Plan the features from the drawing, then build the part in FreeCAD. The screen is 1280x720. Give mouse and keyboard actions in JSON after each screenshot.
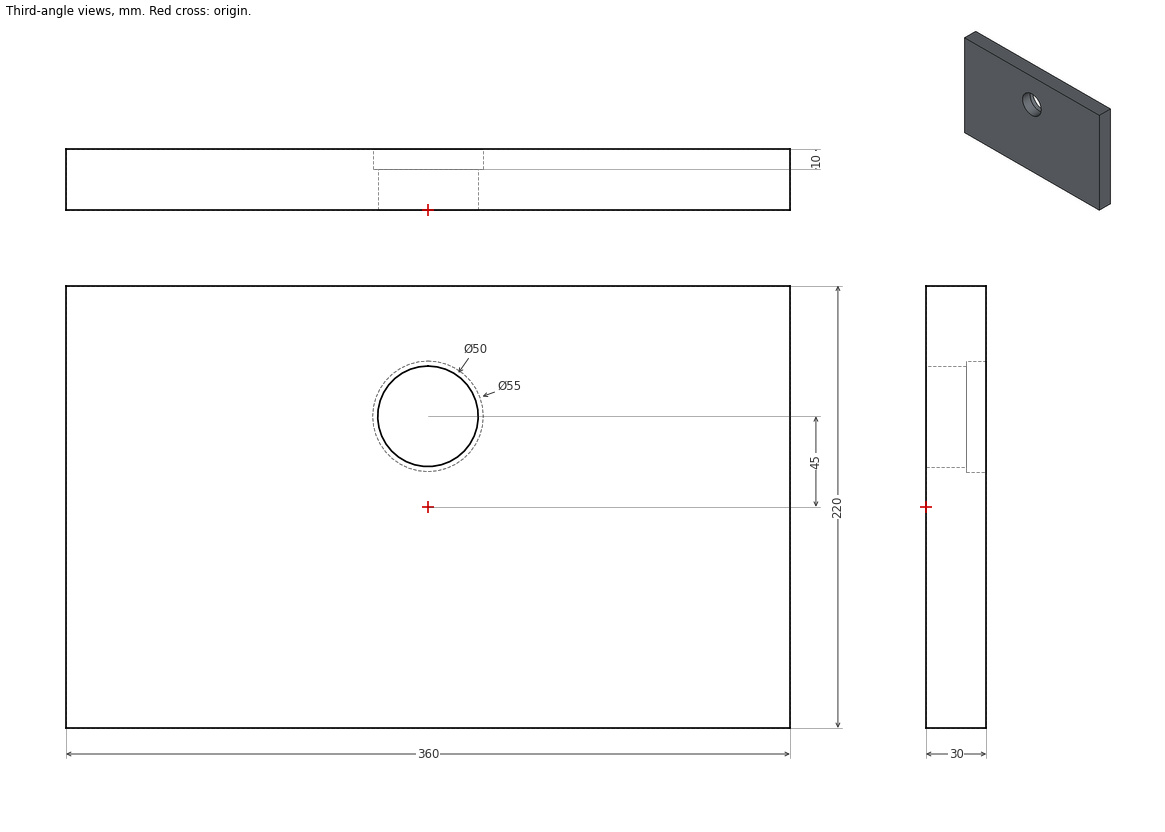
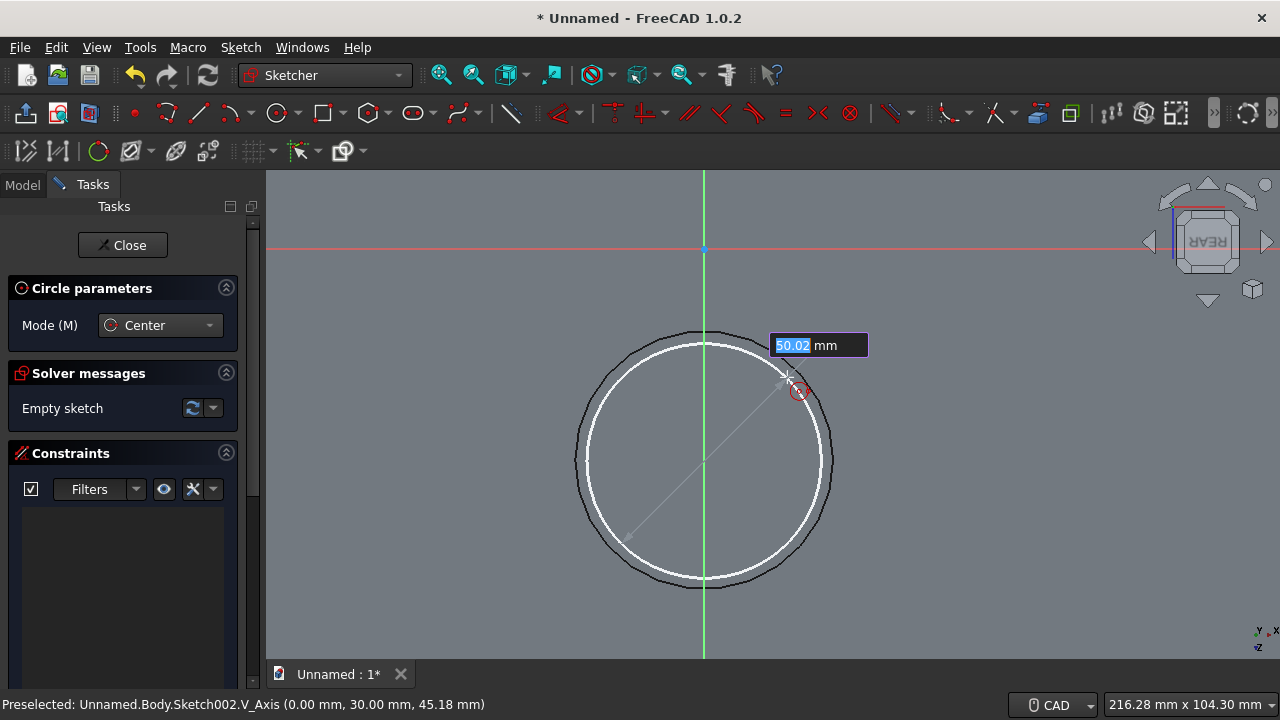
{"action": "type", "text": "50"}
{"action": "key", "text": "Return"}
{"action": "key", "text": "Escape"}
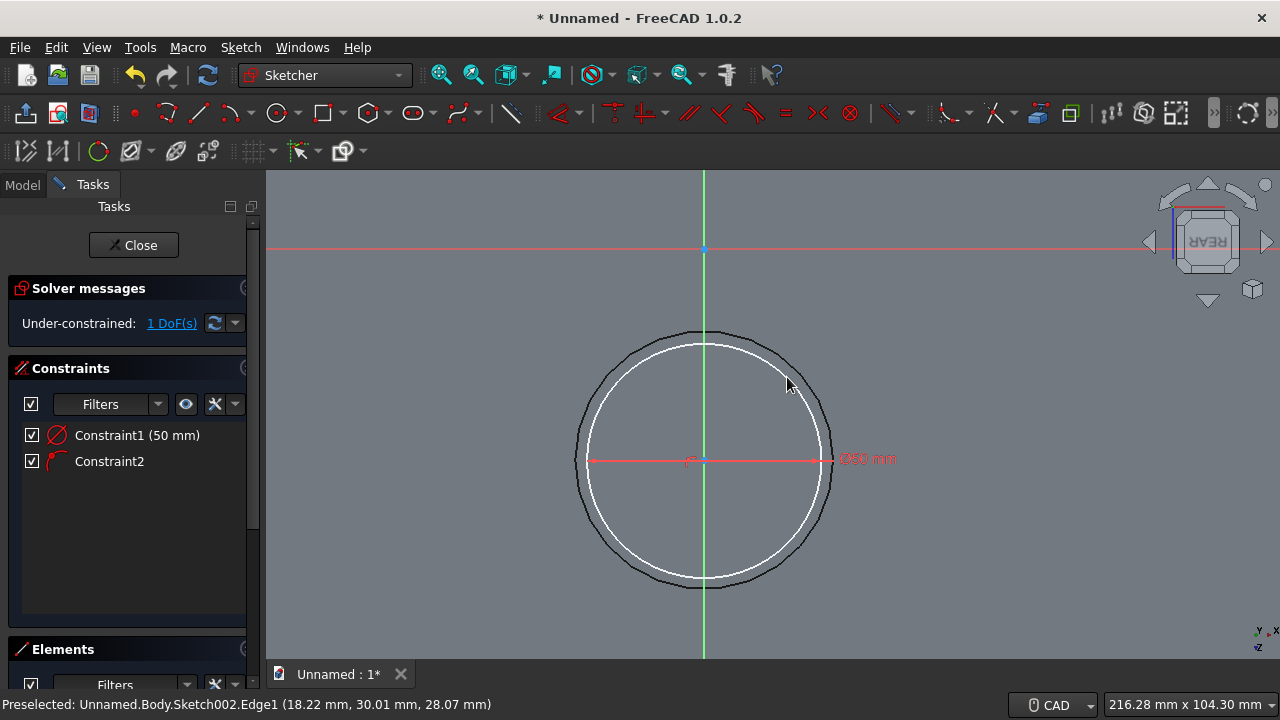
{"action": "key", "text": "d"}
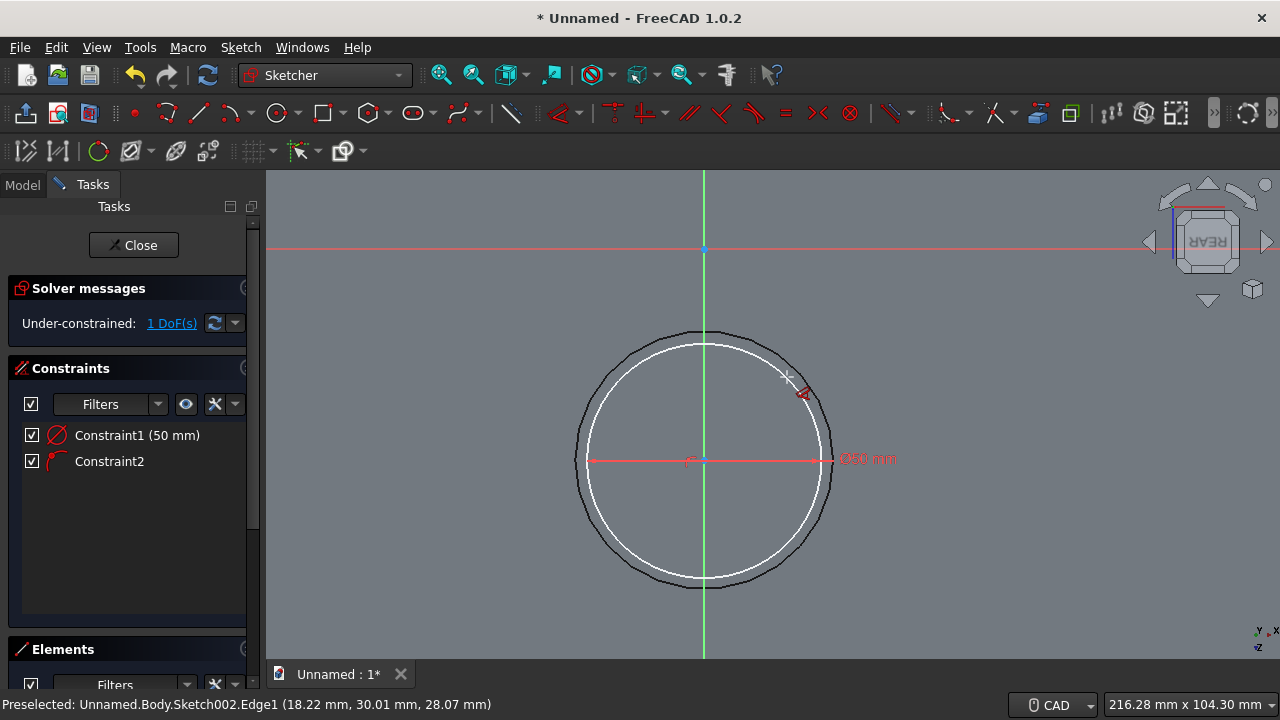
{"action": "left_click", "coordinate": [704, 461]}
{"action": "left_click", "coordinate": [738, 306]}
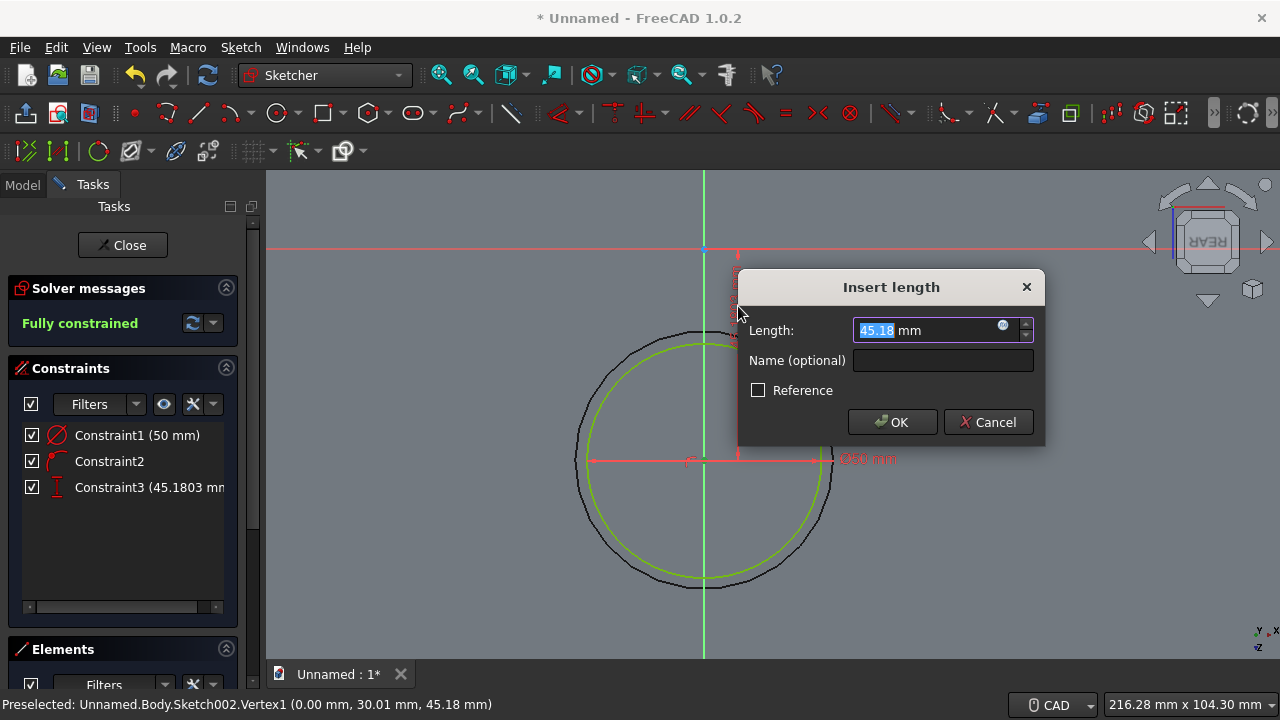
{"action": "type", "text": "45"}
{"action": "key", "text": "Return"}
{"action": "key", "text": "Escape"}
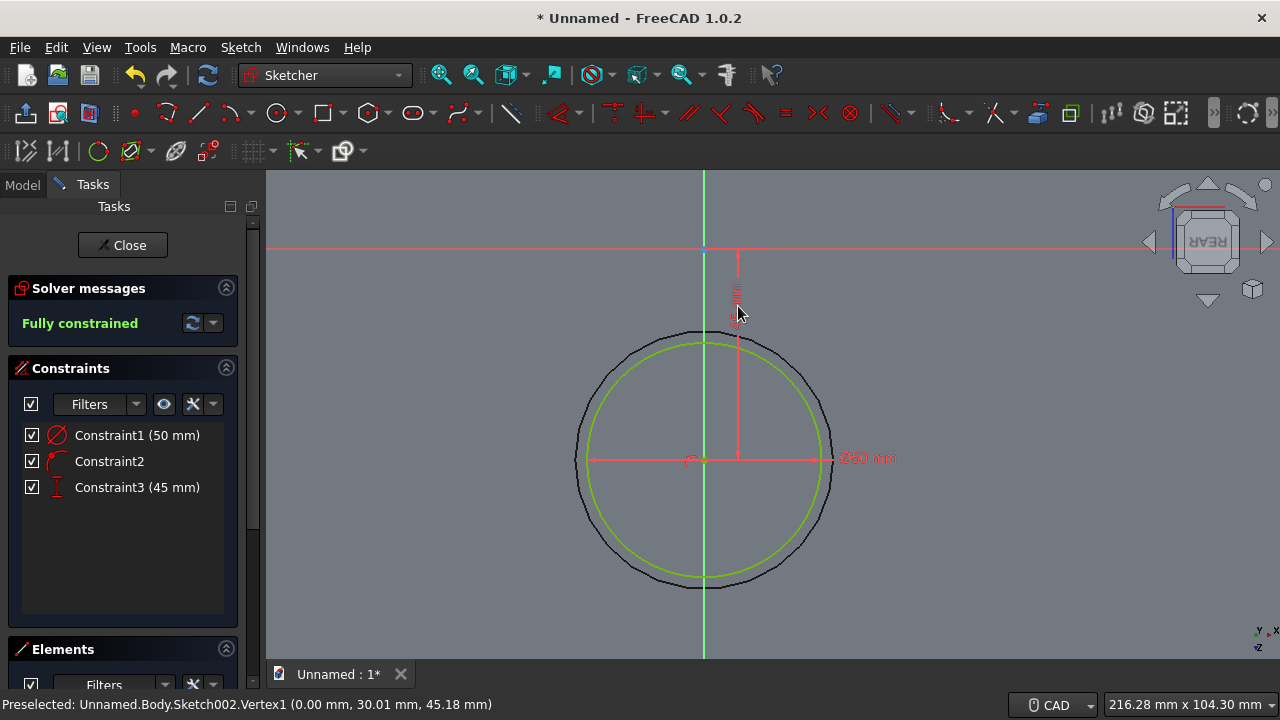
{"action": "left_click", "coordinate": [123, 245]}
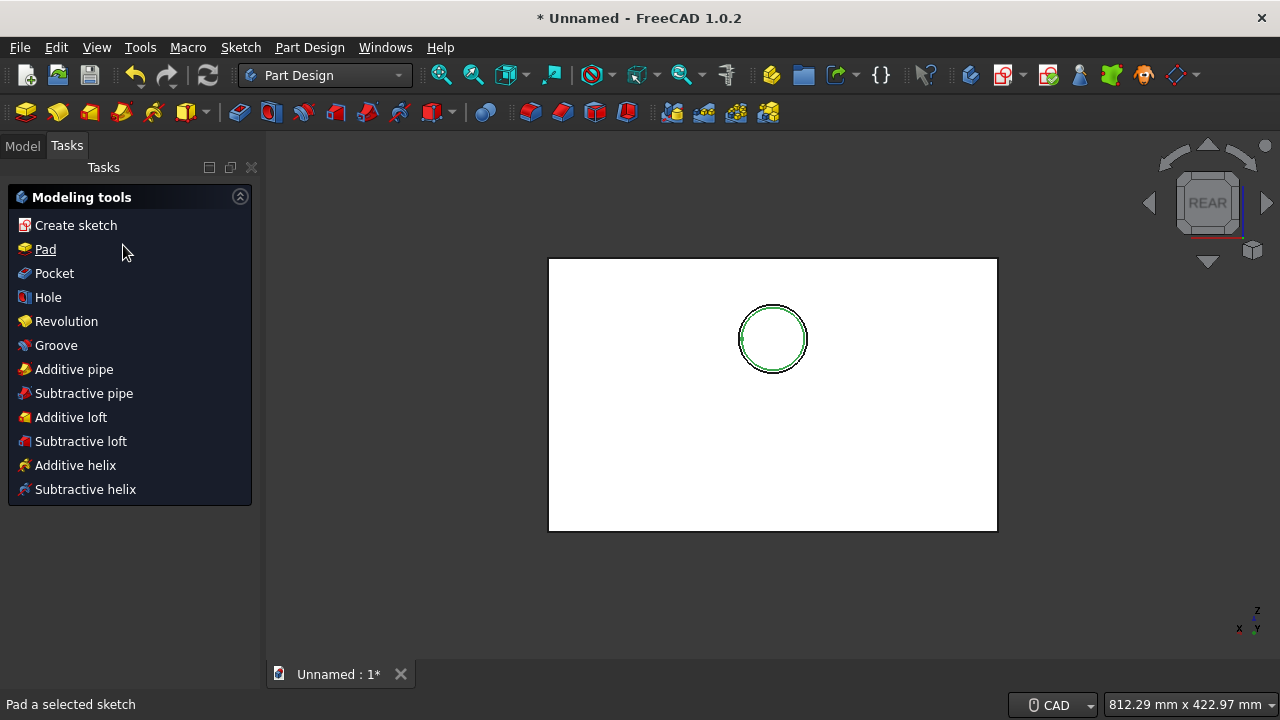
{"action": "left_click", "coordinate": [240, 112]}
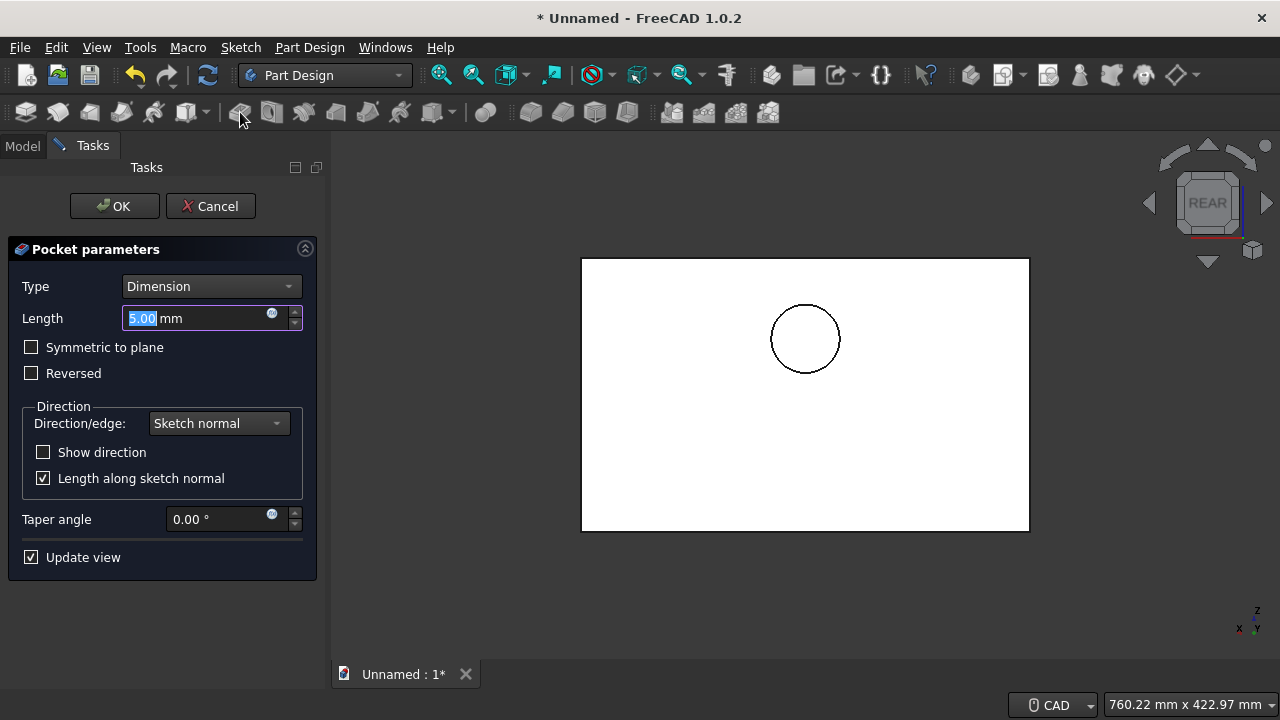
{"action": "left_click", "coordinate": [212, 286]}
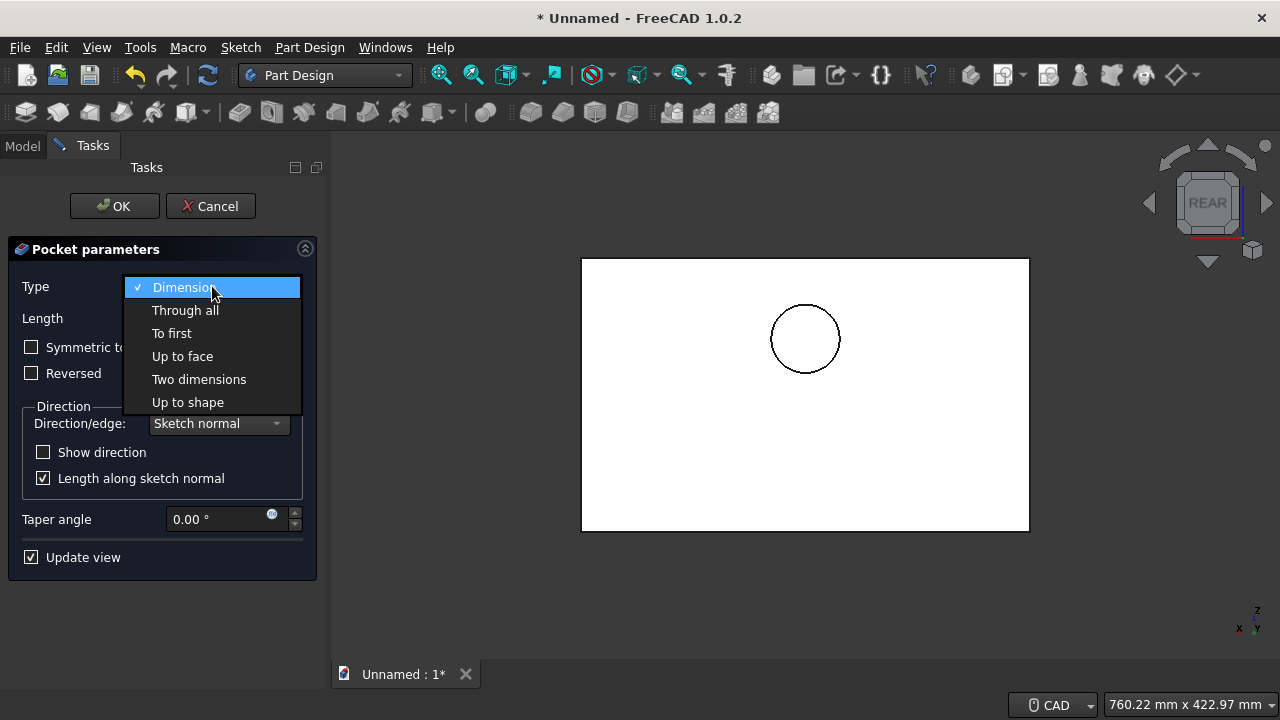
{"action": "left_click", "coordinate": [212, 310]}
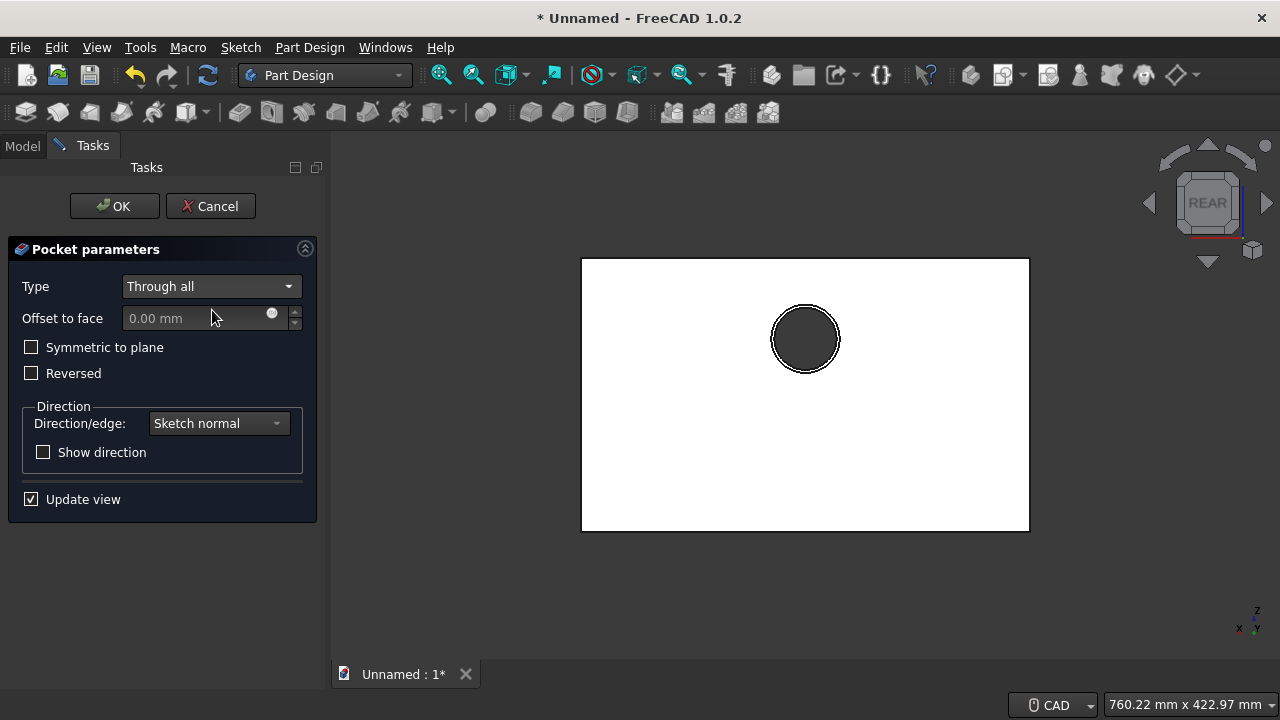
{"action": "left_click", "coordinate": [115, 206]}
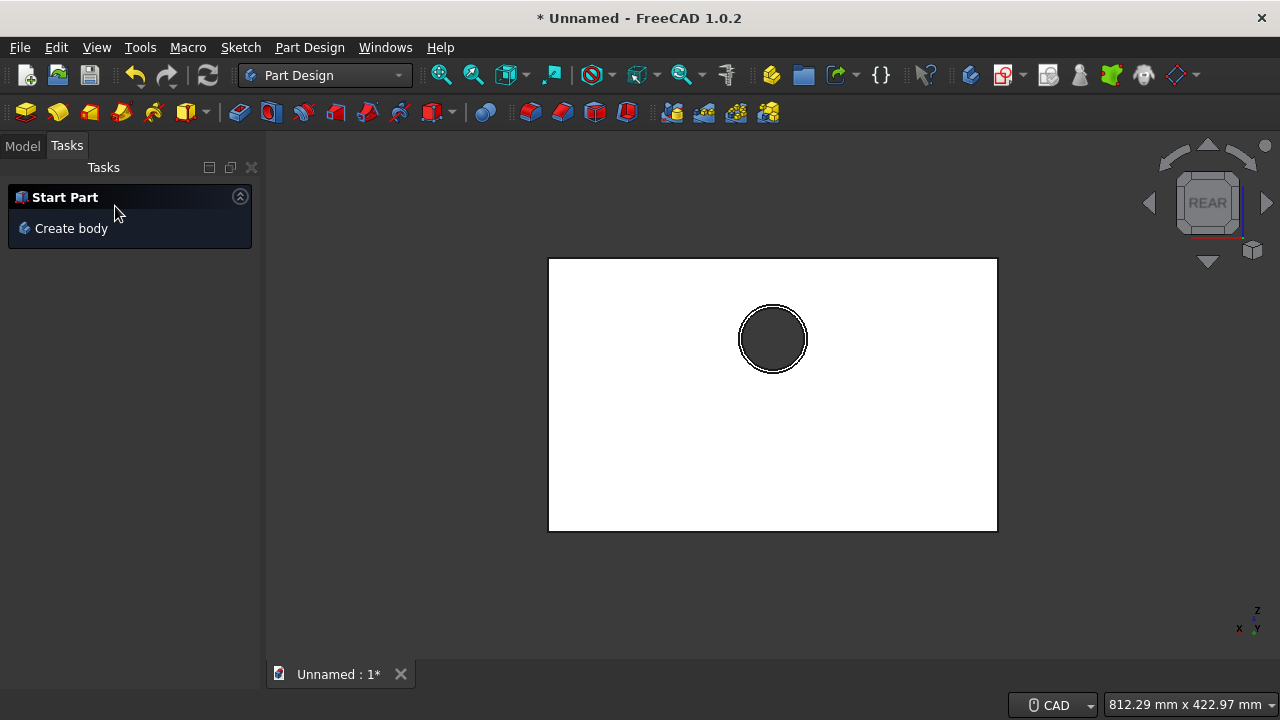
{"action": "key", "text": "0"}